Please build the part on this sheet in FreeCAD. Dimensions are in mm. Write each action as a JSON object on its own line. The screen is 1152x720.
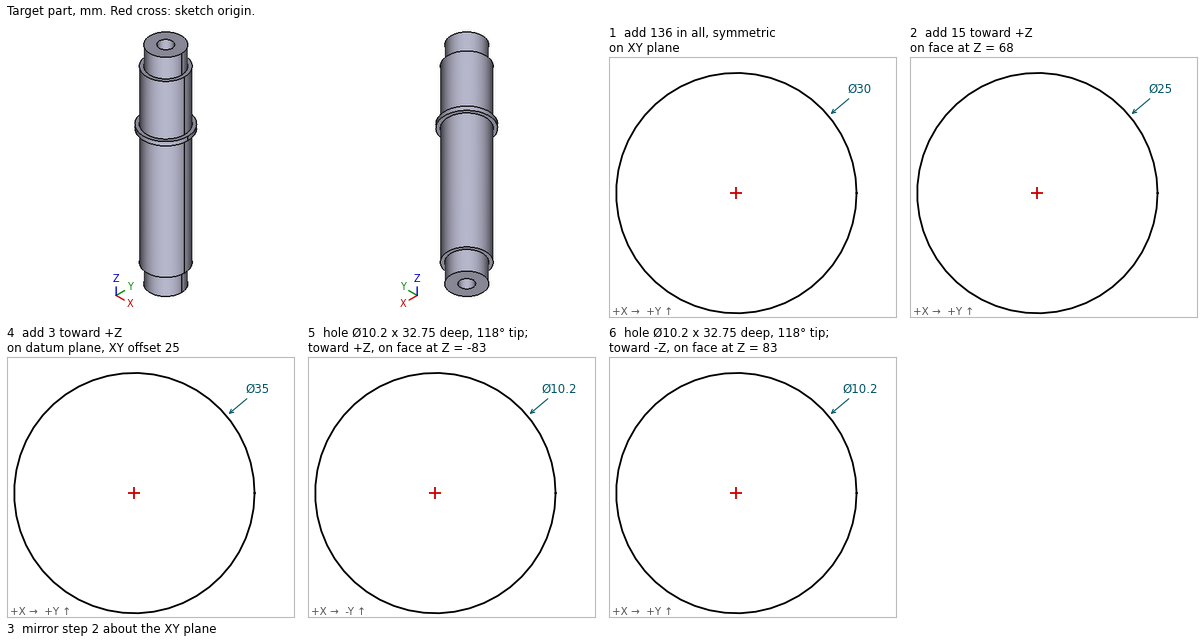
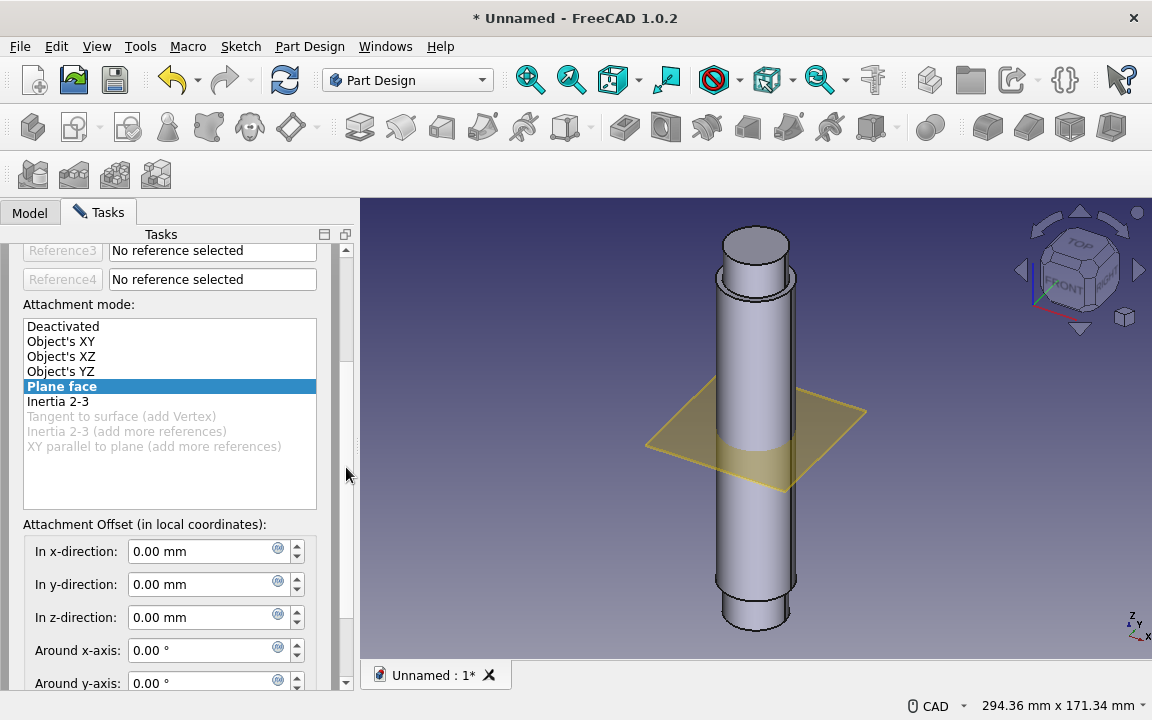
{"action": "triple_click", "coordinate": [210, 558]}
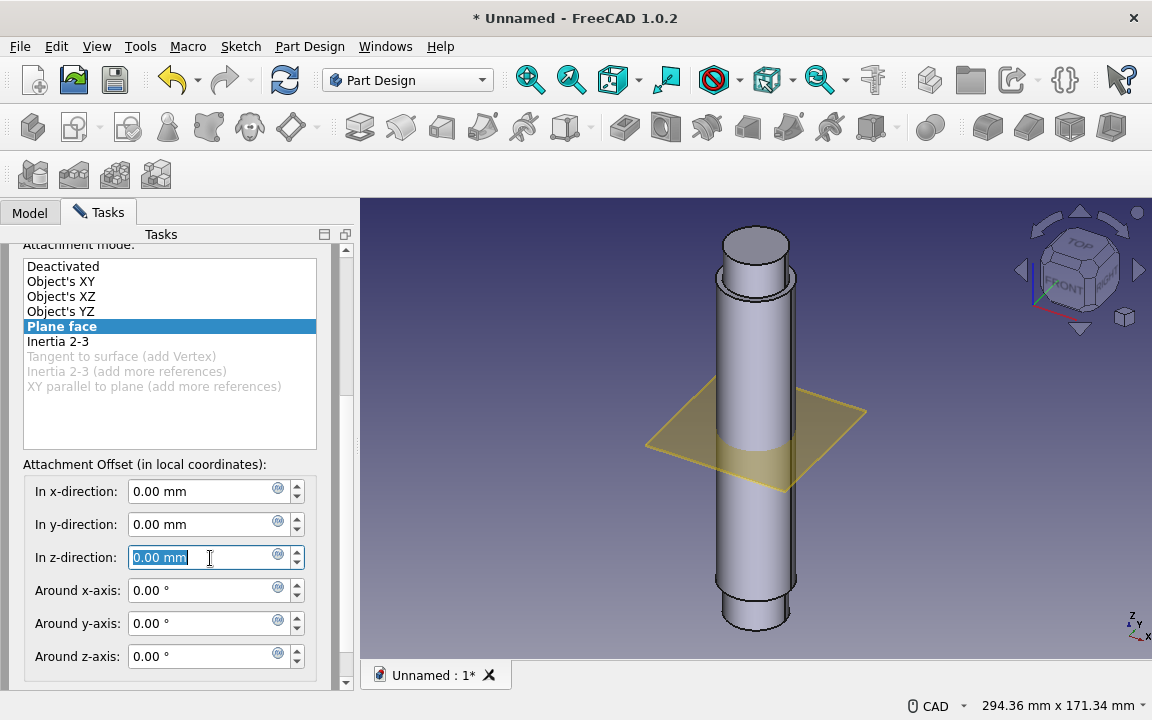
{"action": "type", "text": "25"}
{"action": "key", "text": "Tab"}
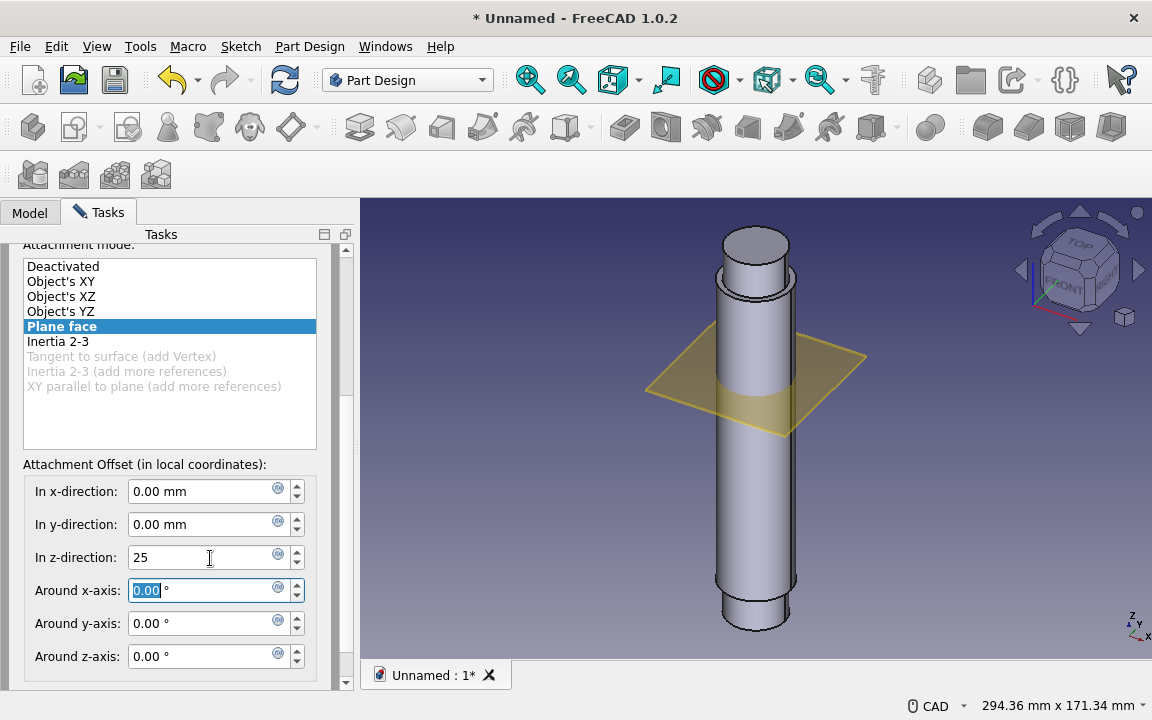
{"action": "scroll", "coordinate": [346, 467], "scroll_direction": "up", "scroll_amount": 5}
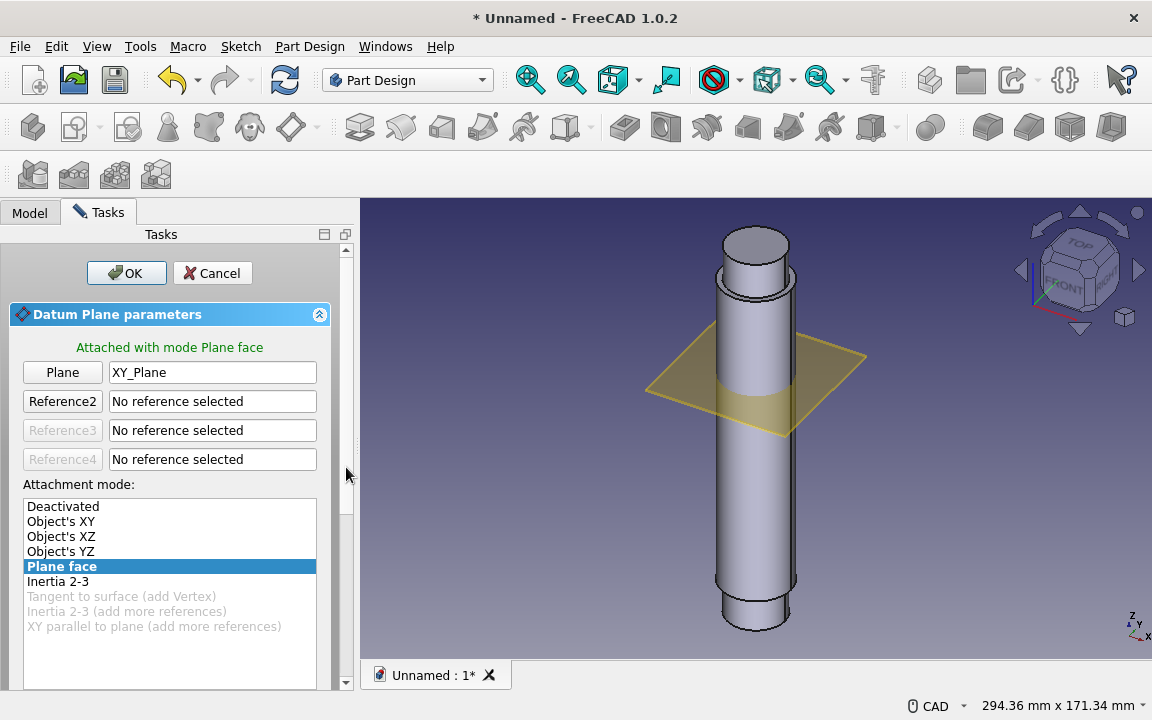
{"action": "left_click", "coordinate": [127, 273]}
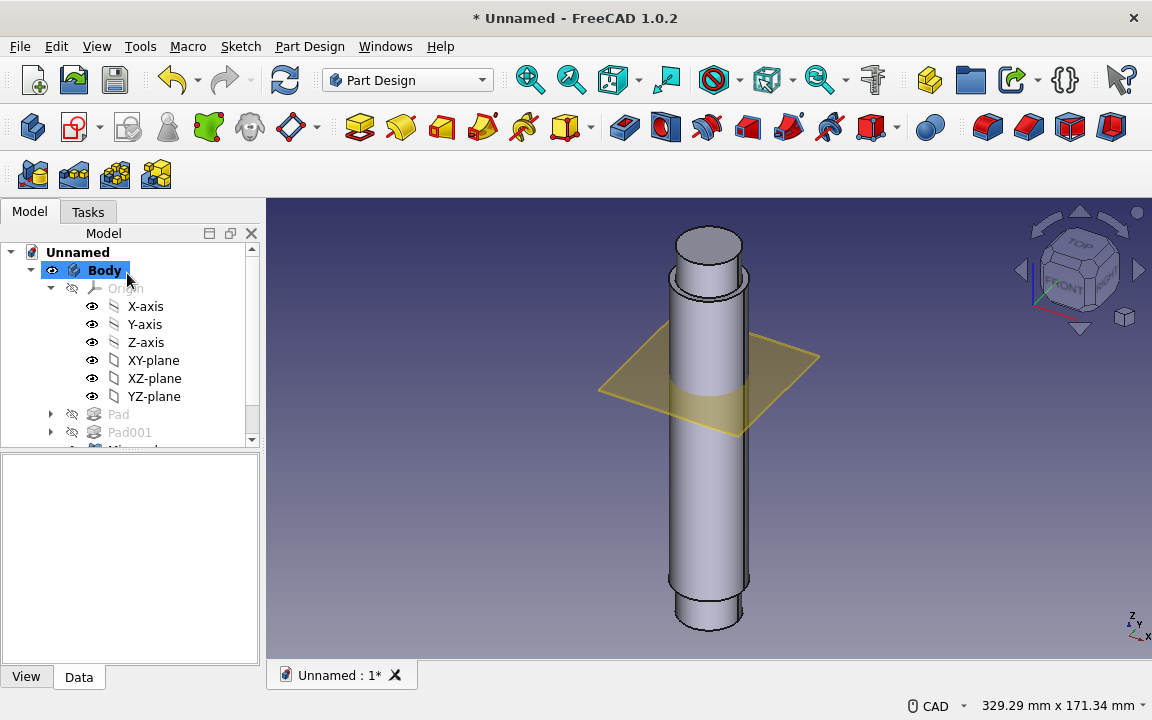
{"action": "scroll", "coordinate": [101, 338], "scroll_direction": "down", "scroll_amount": 3}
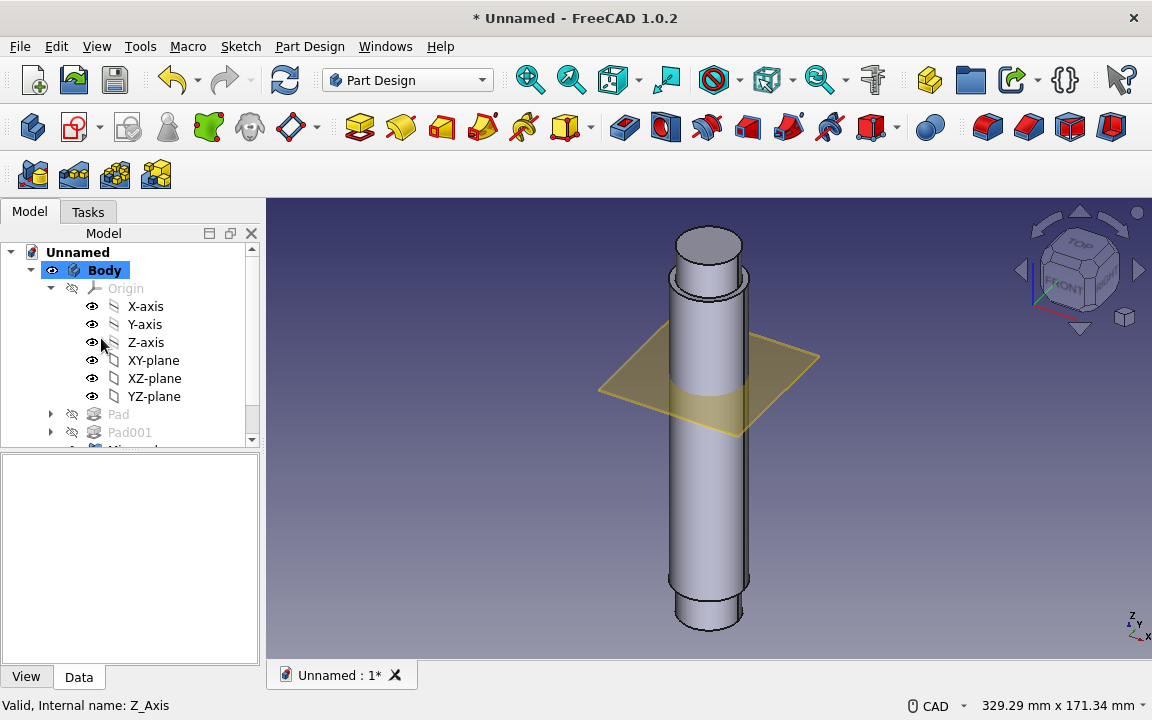
{"action": "left_click", "coordinate": [117, 432]}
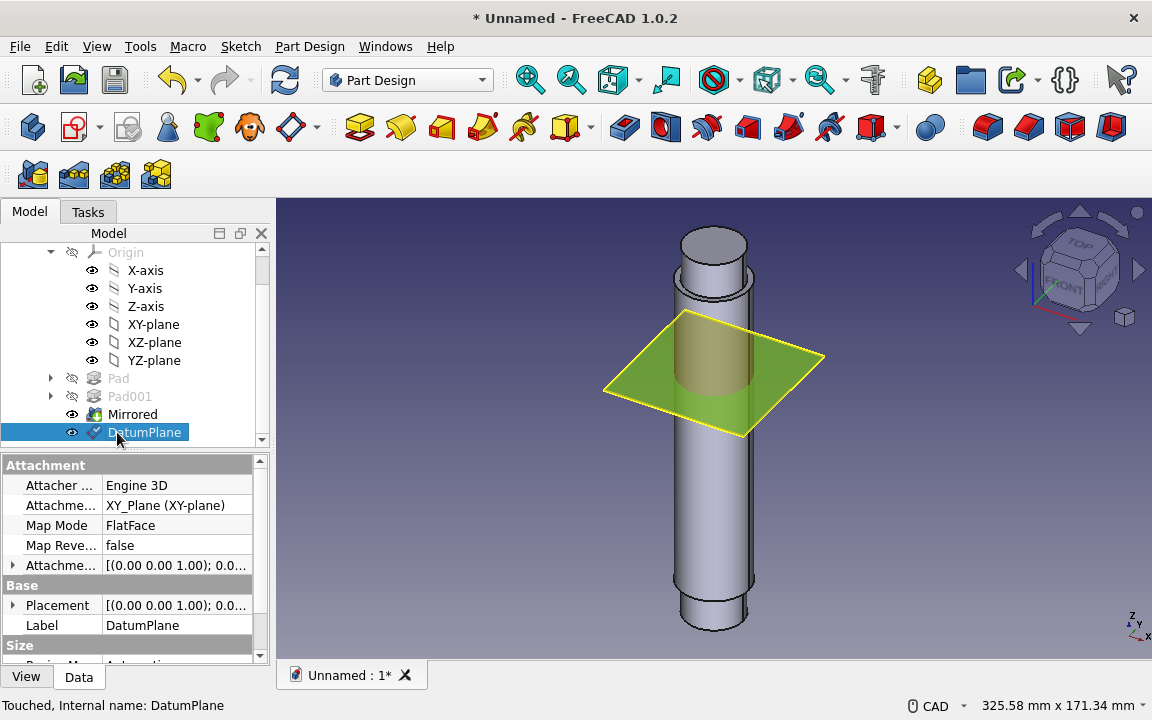
{"action": "left_click", "coordinate": [74, 128]}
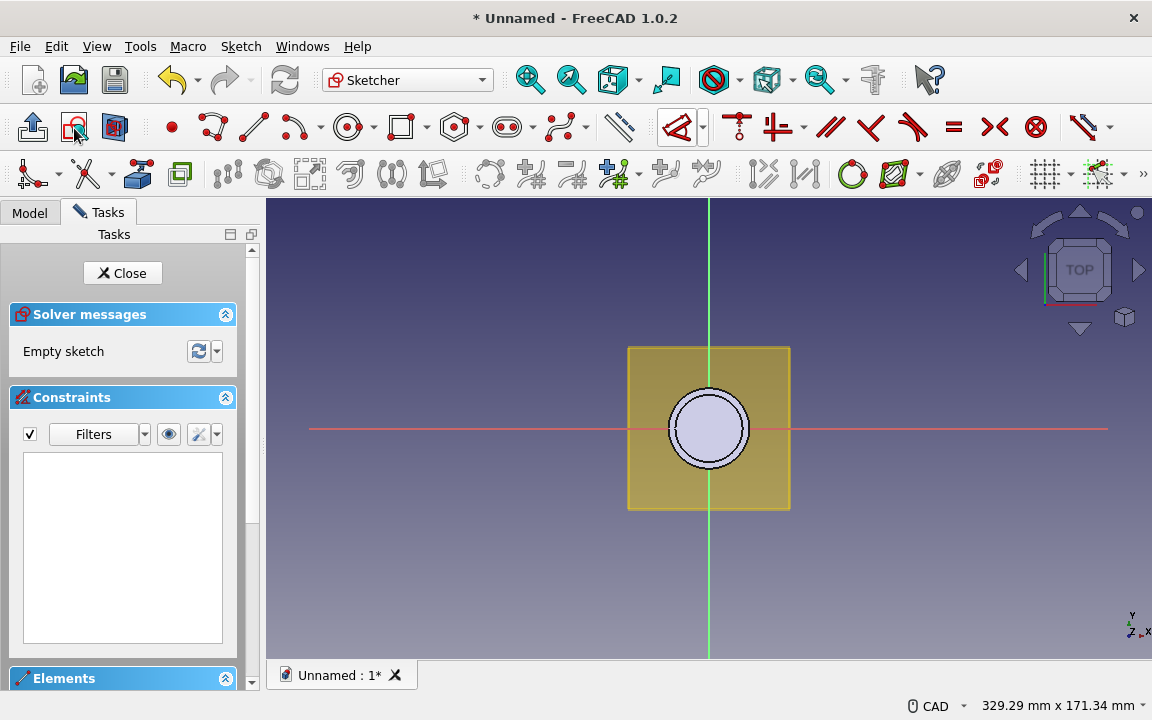
{"action": "left_click", "coordinate": [115, 128]}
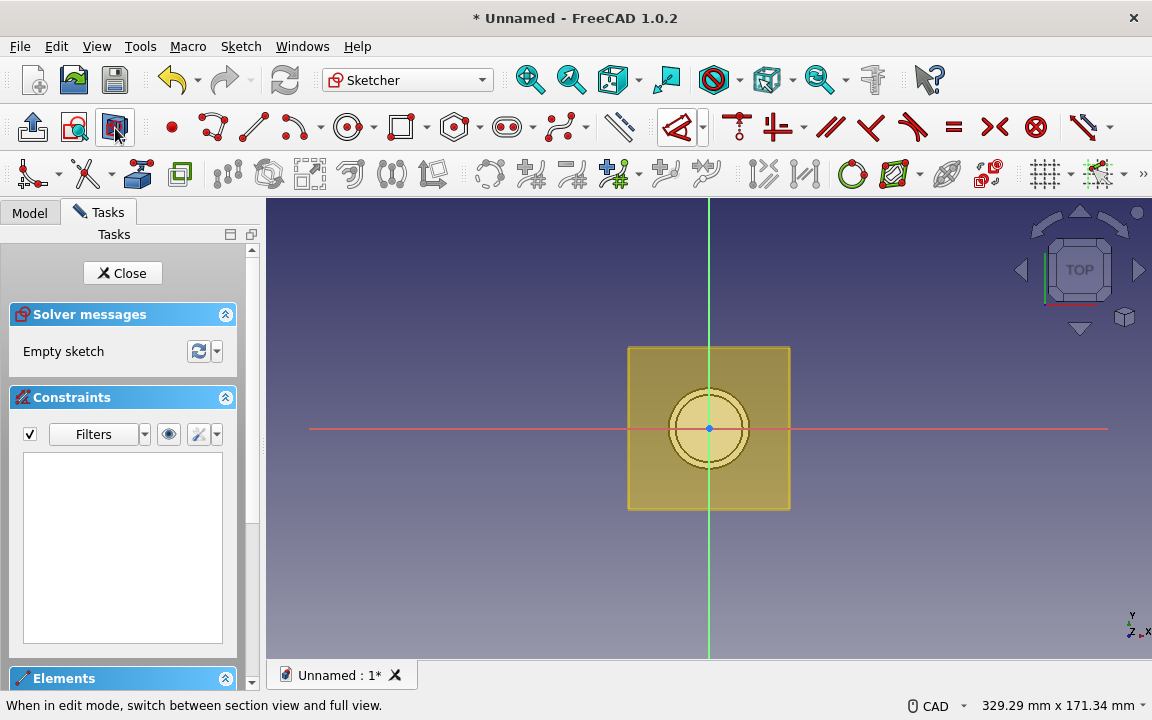
{"action": "scroll", "coordinate": [739, 428], "scroll_direction": "up", "scroll_amount": 6}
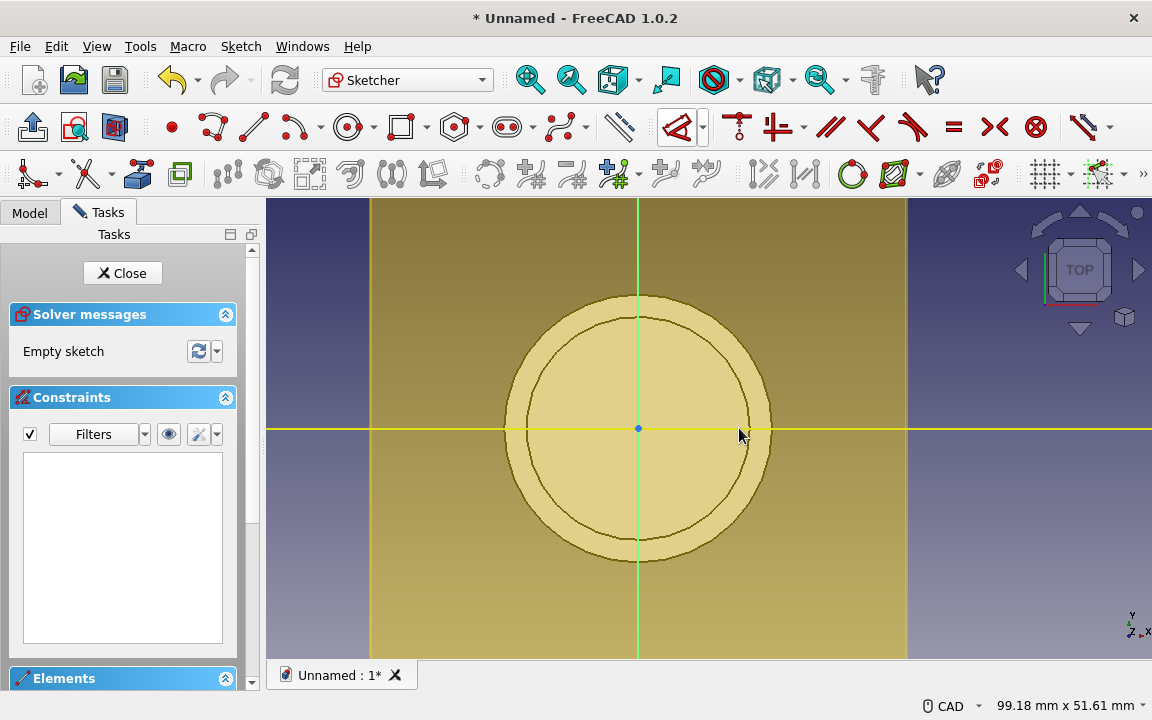
{"action": "left_click", "coordinate": [348, 128]}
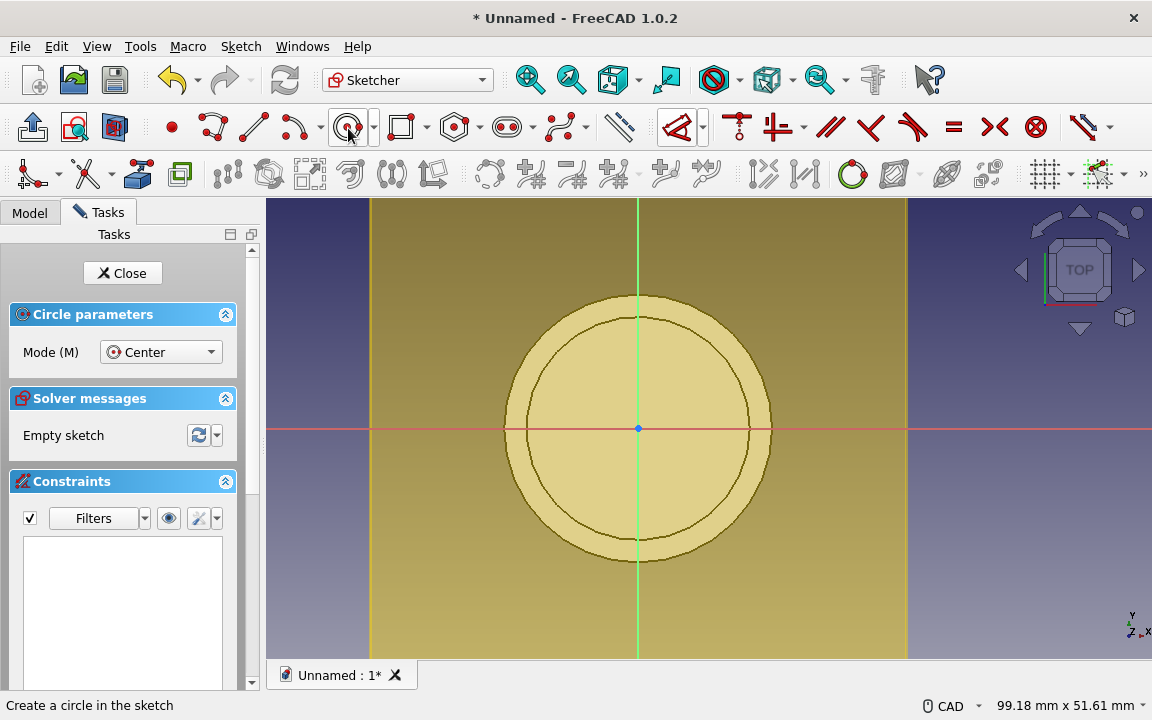
{"action": "left_click", "coordinate": [638, 428]}
{"action": "mouse_move", "coordinate": [749, 318]}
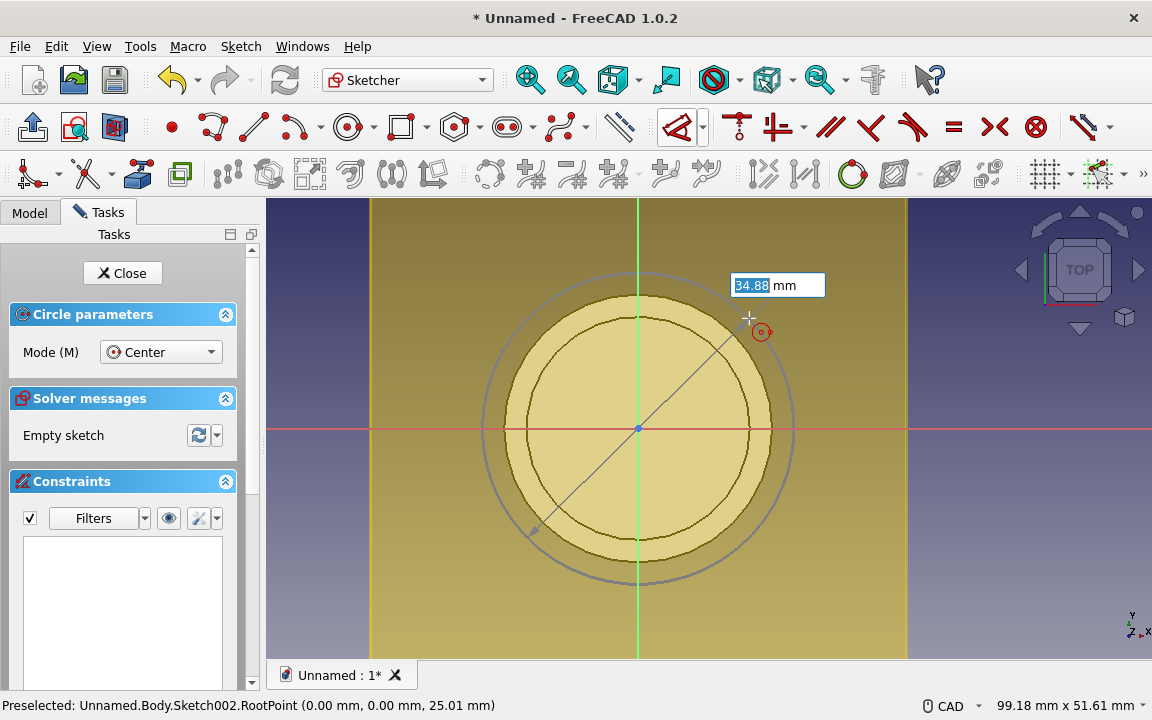
{"action": "type", "text": "35"}
{"action": "key", "text": "Return"}
{"action": "key", "text": "Escape"}